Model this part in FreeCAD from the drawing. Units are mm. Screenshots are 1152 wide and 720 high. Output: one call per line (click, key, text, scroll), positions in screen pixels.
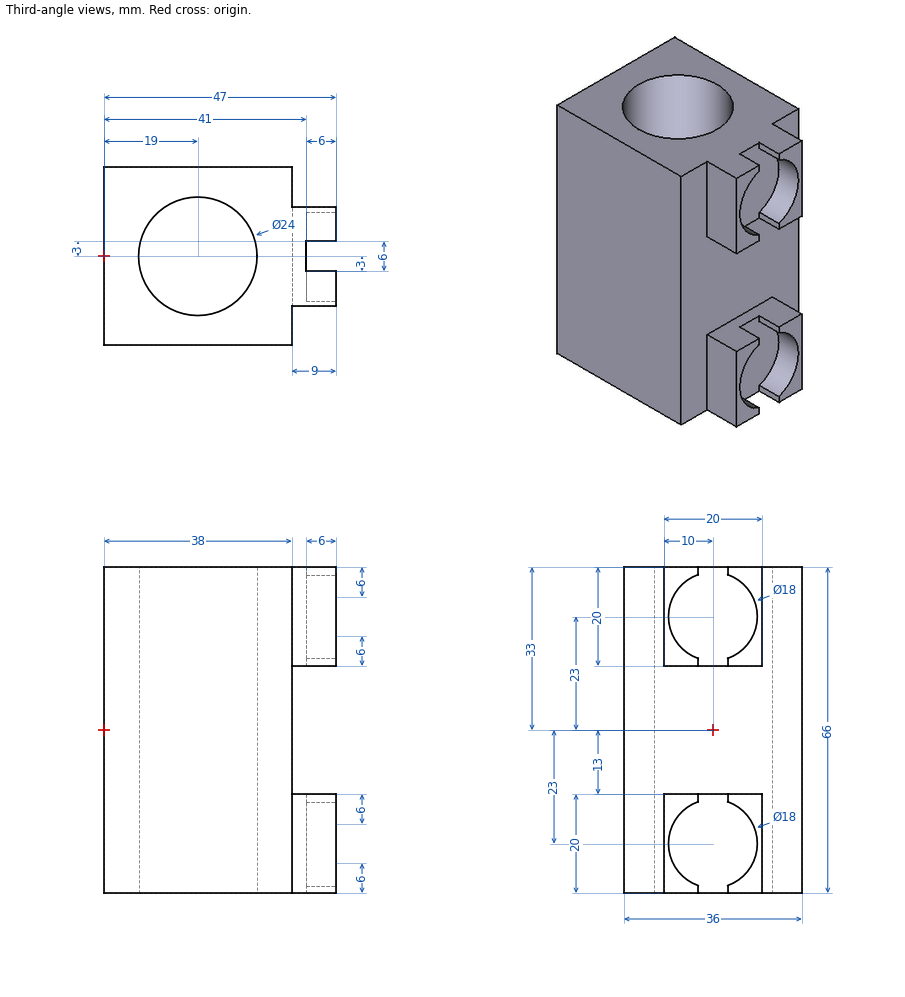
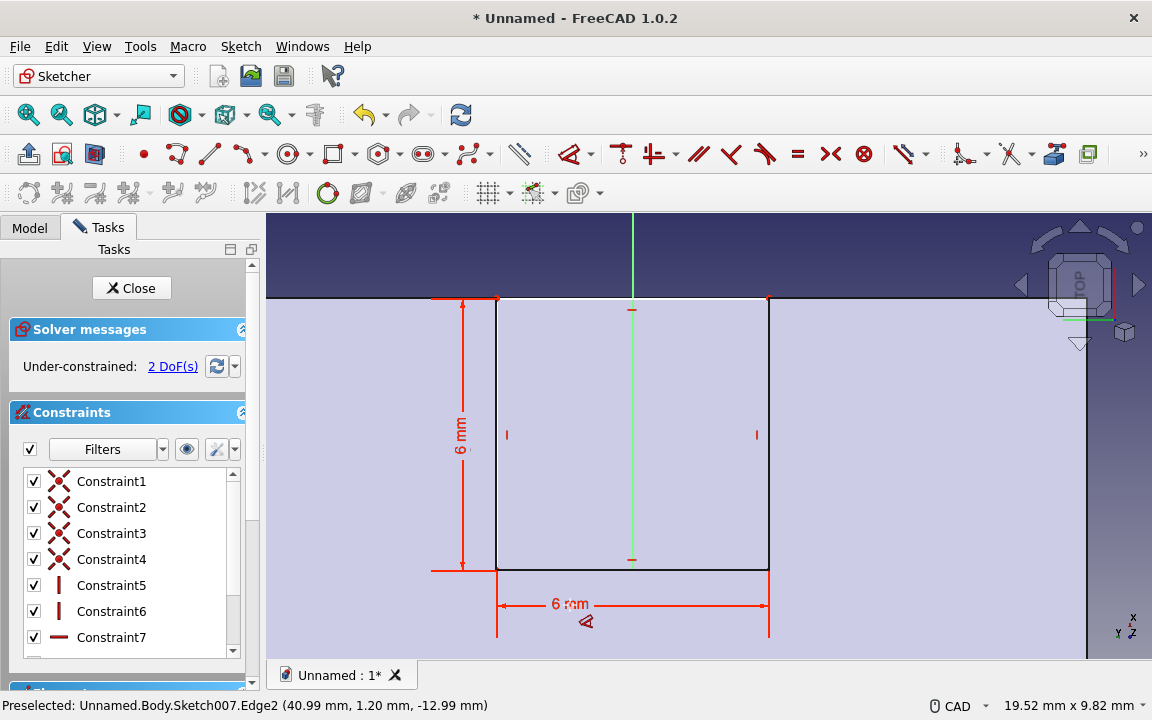
click(497, 299)
click(565, 265)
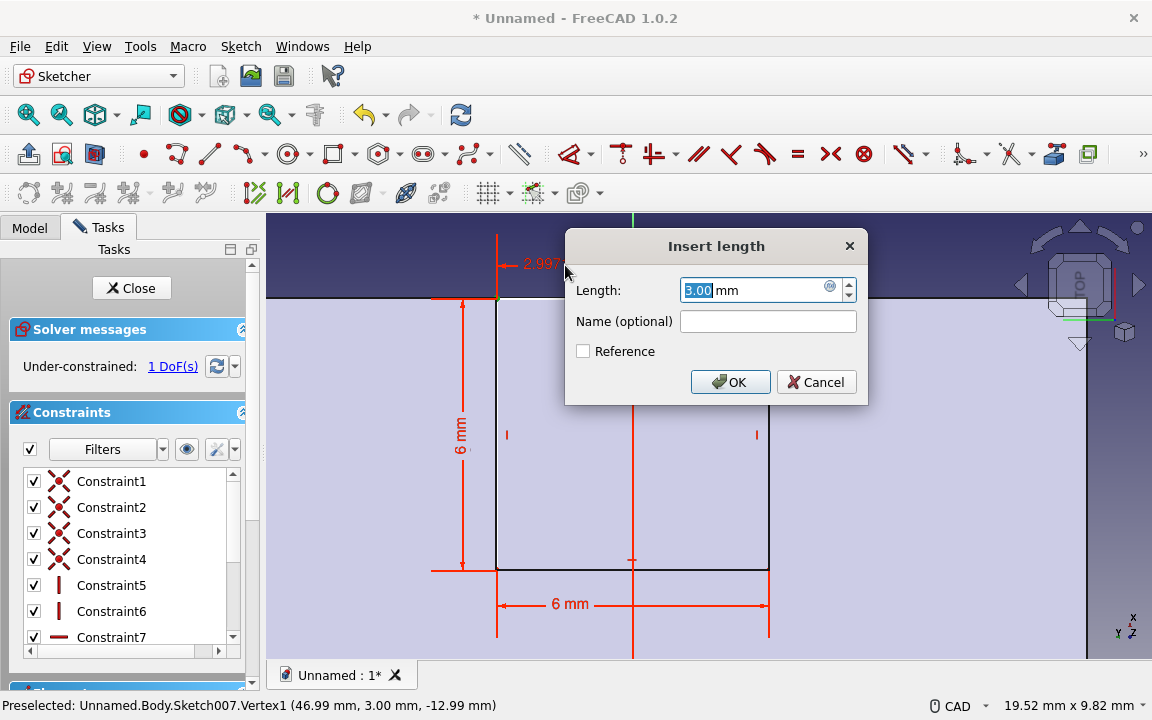
text(3)
key(Return)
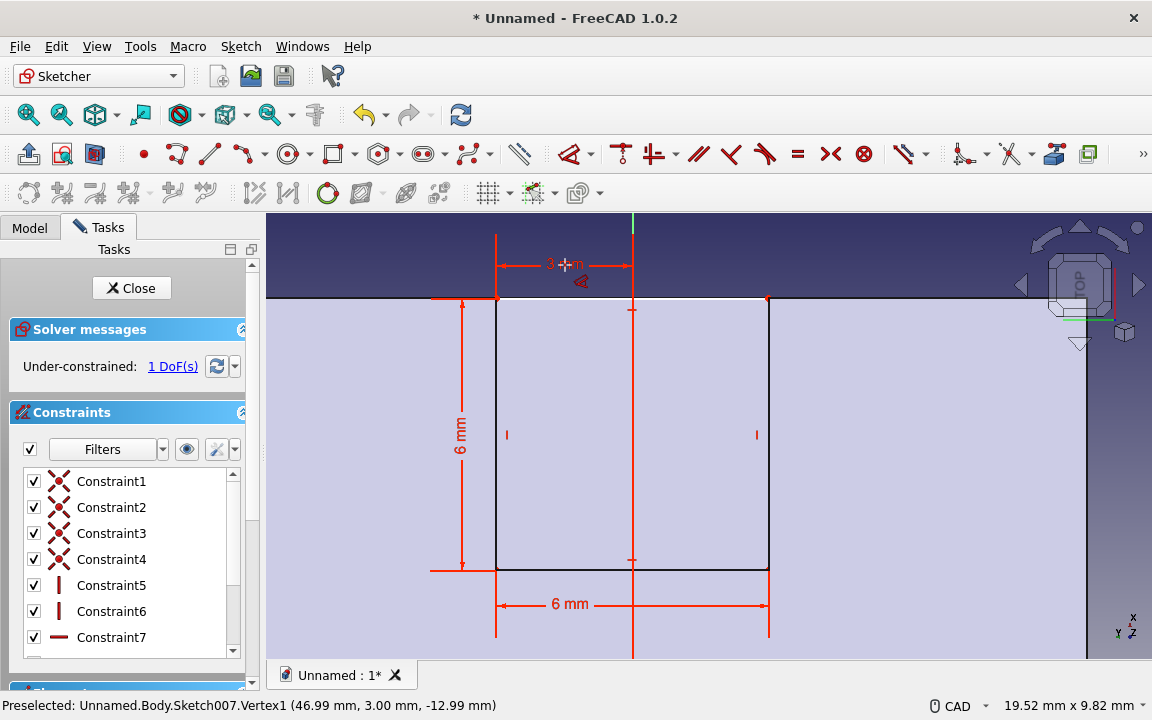
click(496, 299)
click(462, 465)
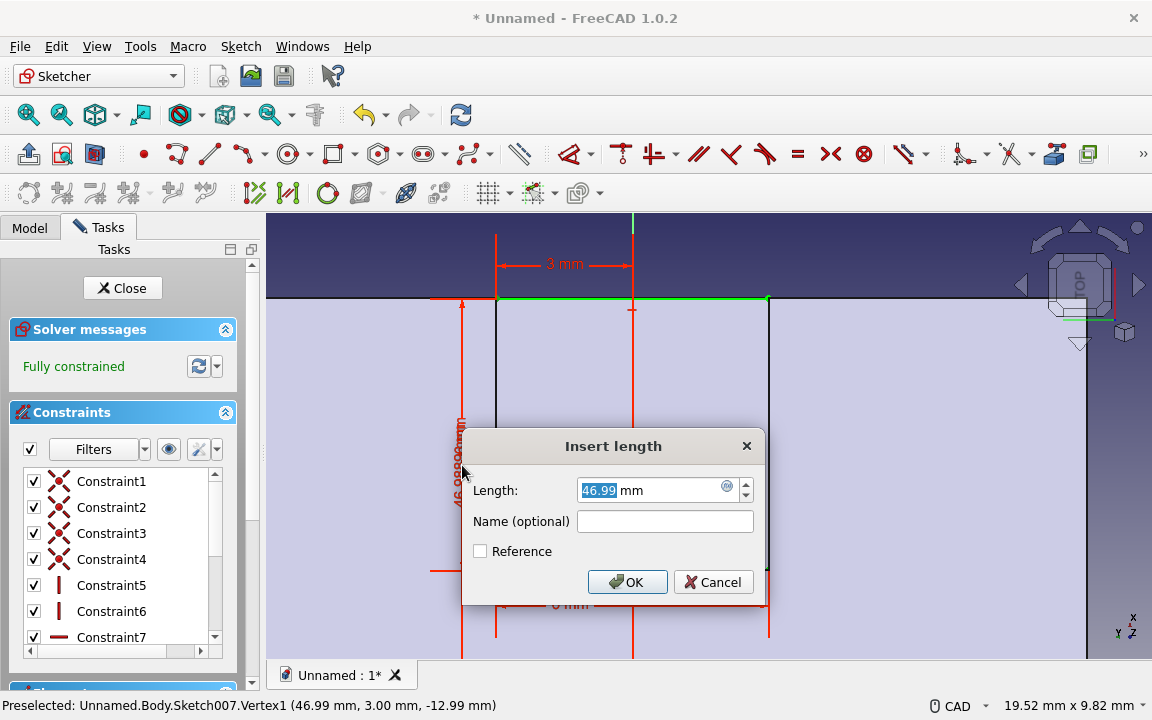
text(47)
key(Return)
key(Escape)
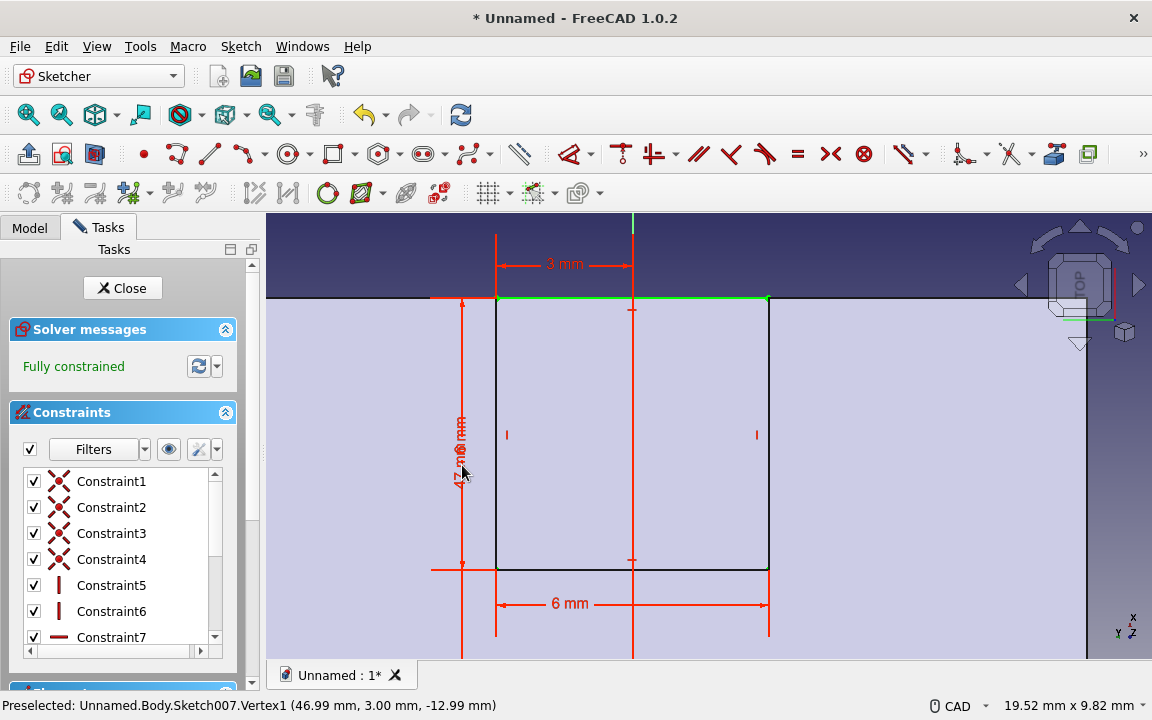
click(123, 288)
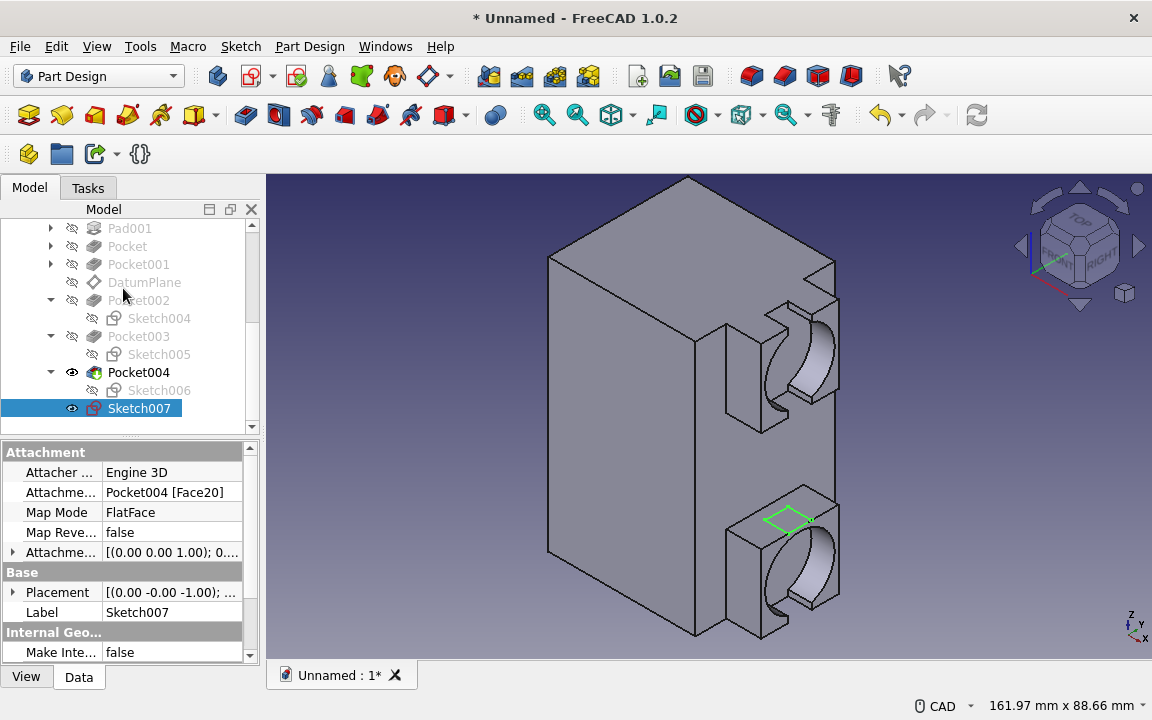
click(246, 116)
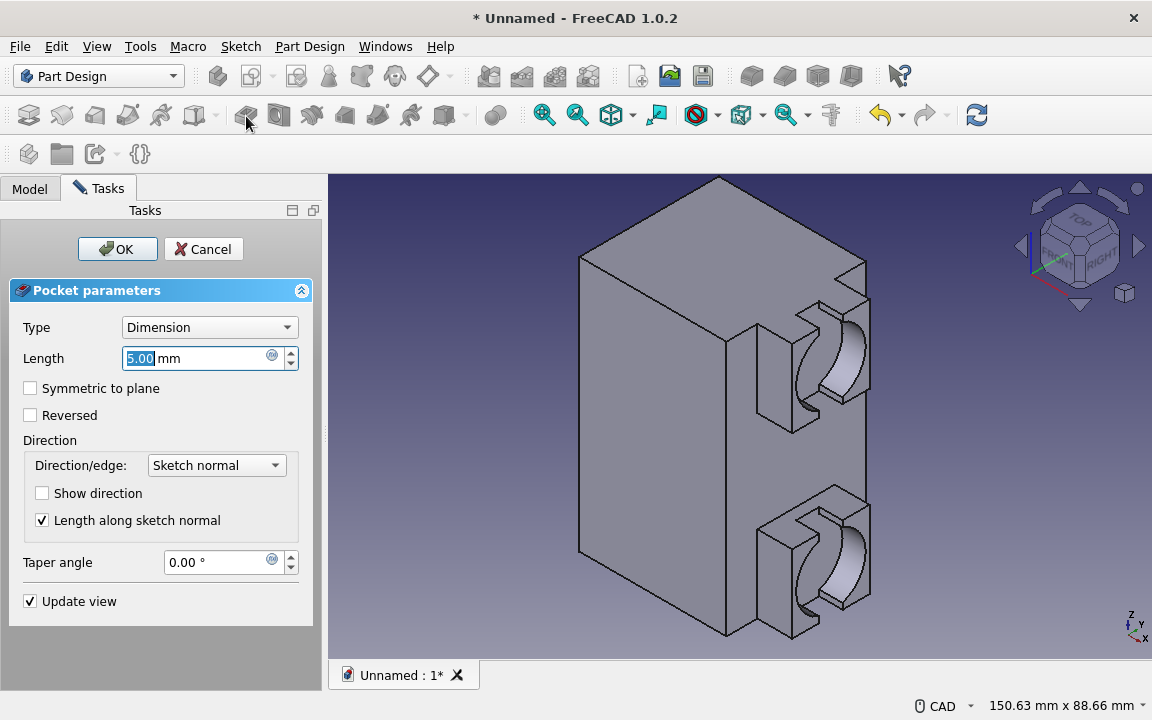
text(6)
key(Tab)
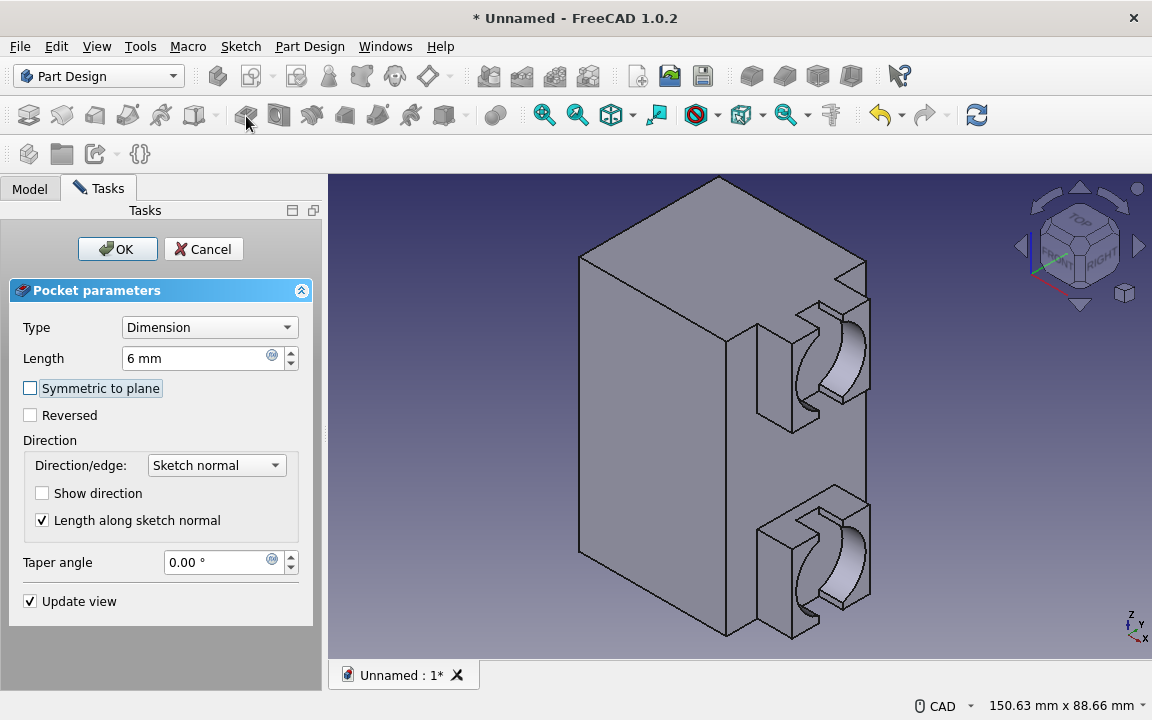
click(118, 249)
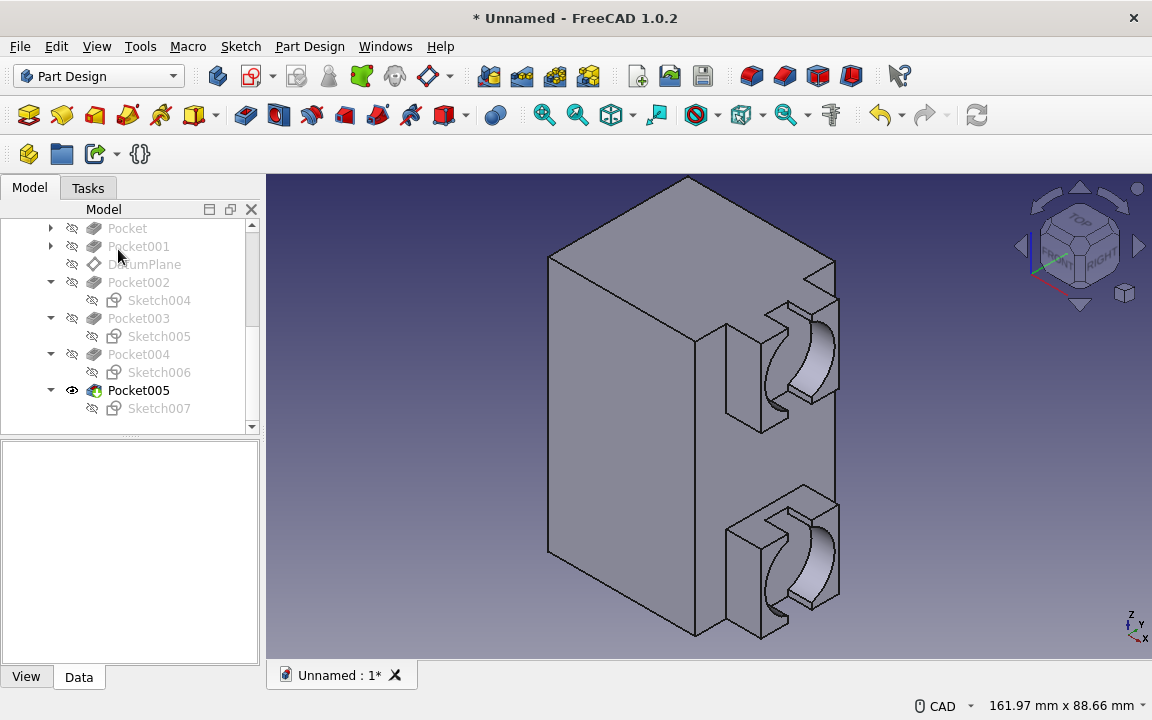
click(709, 268)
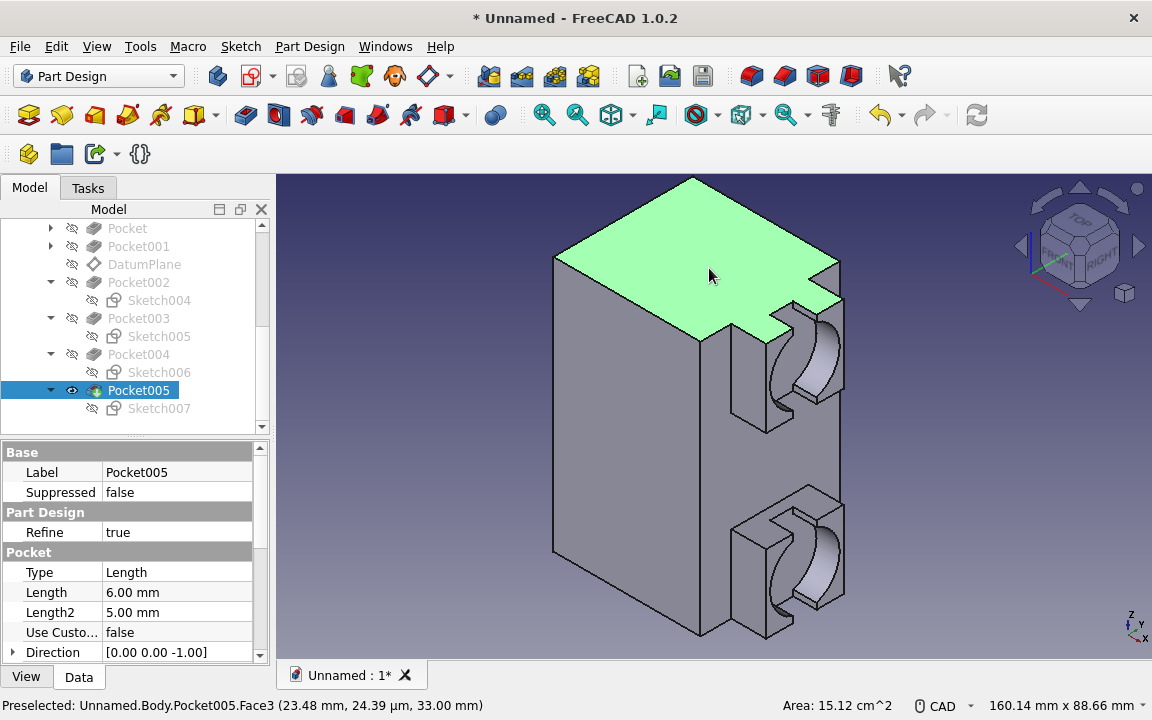
click(250, 76)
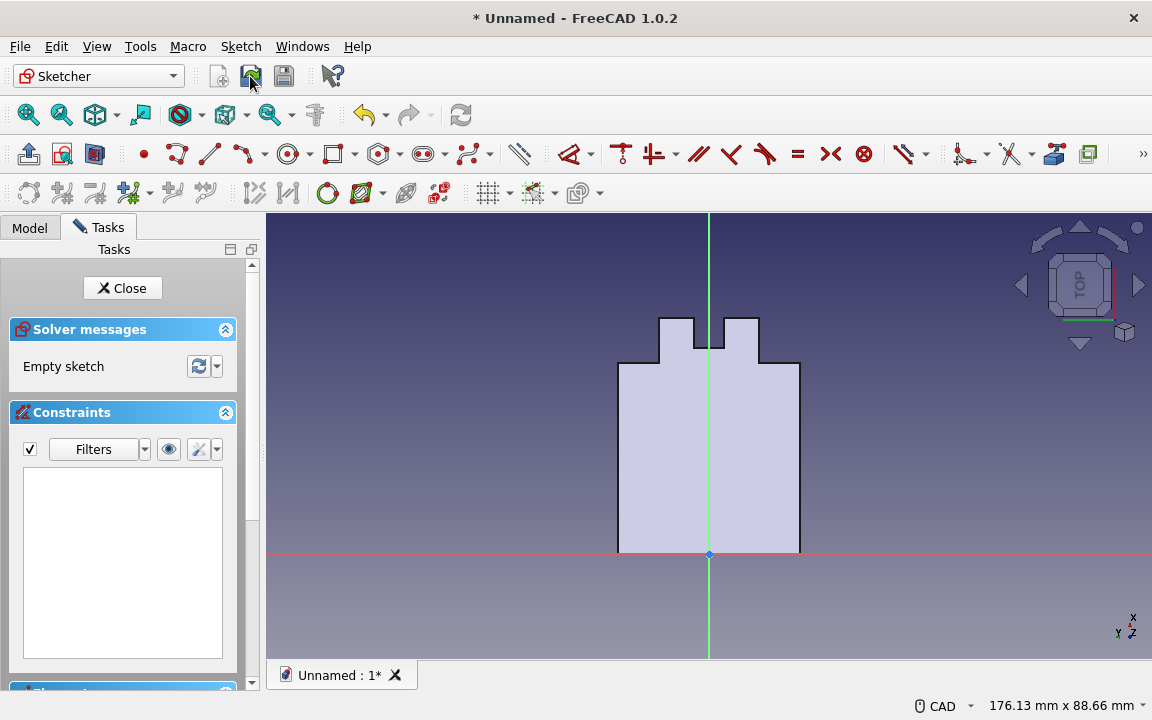
scroll(792, 525, up, 3)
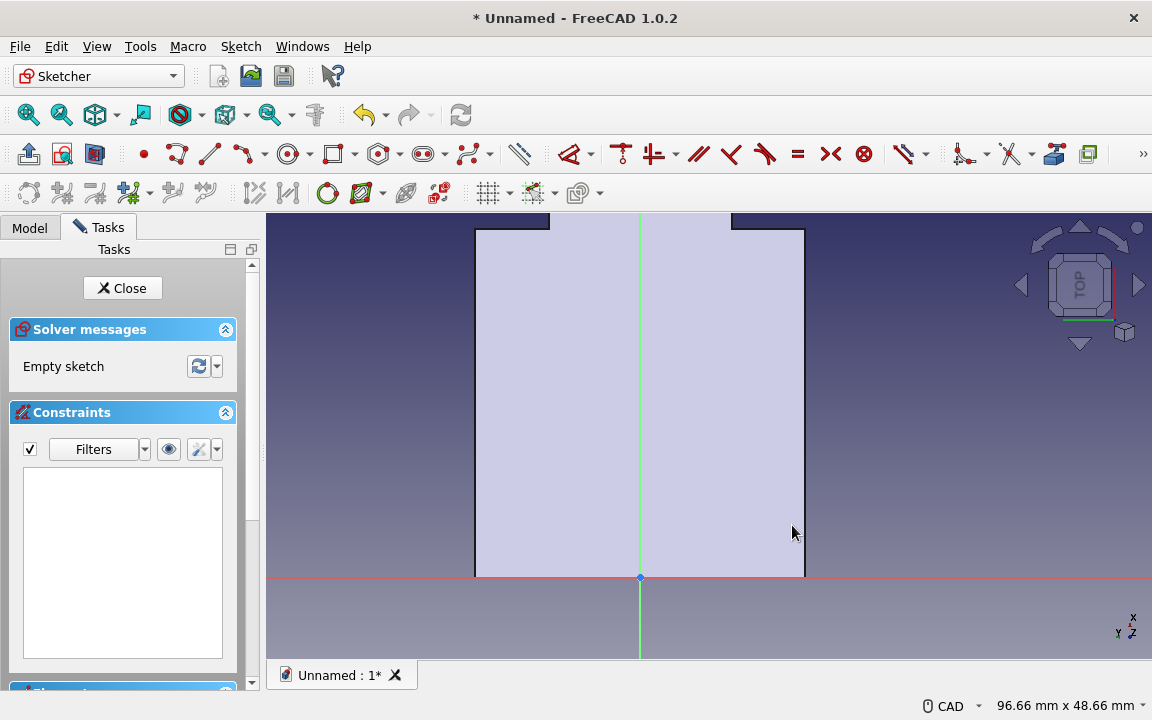
click(288, 154)